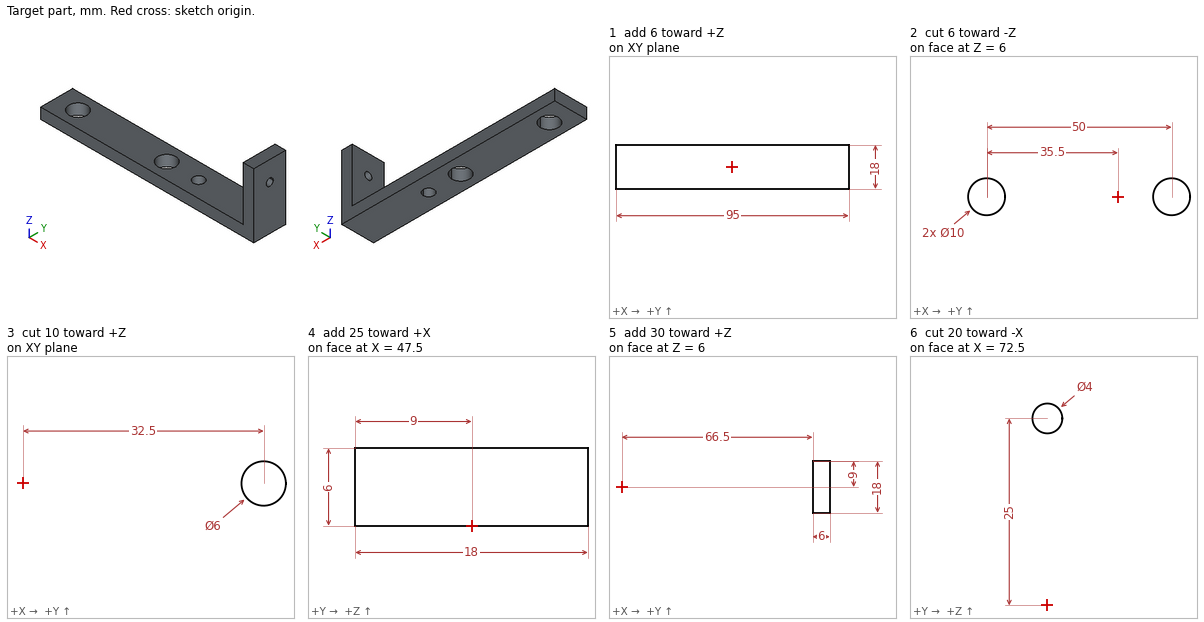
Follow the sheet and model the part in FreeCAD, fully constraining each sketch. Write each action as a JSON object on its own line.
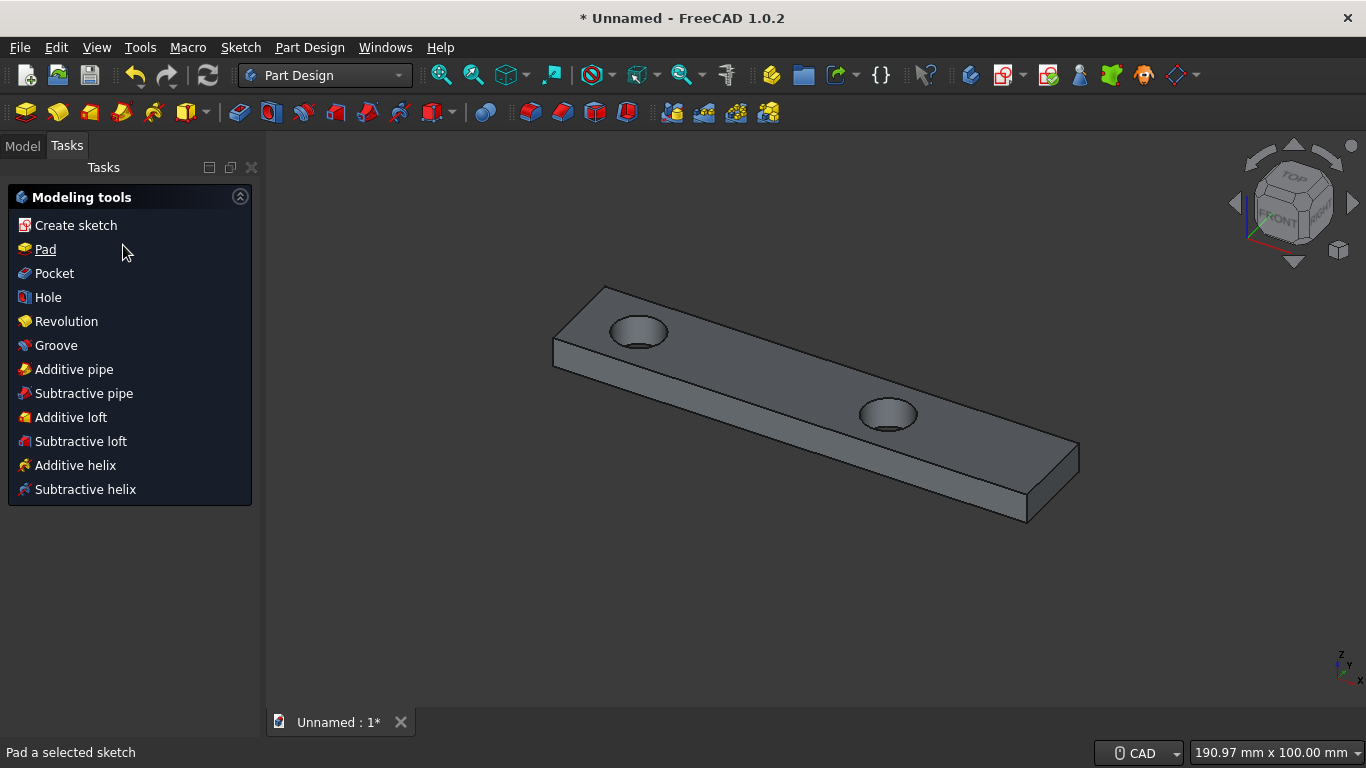
{"action": "left_click", "coordinate": [240, 112]}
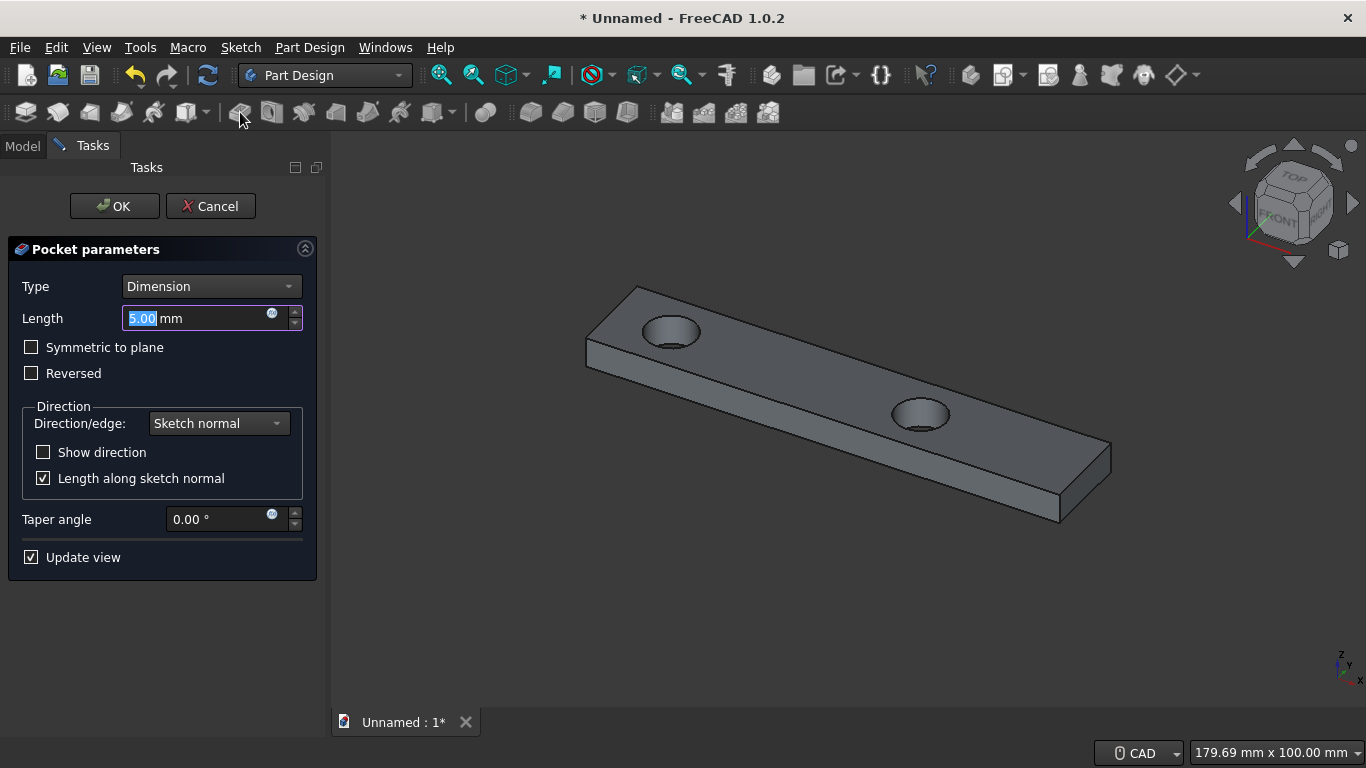
{"action": "type", "text": "10"}
{"action": "key", "text": "Tab"}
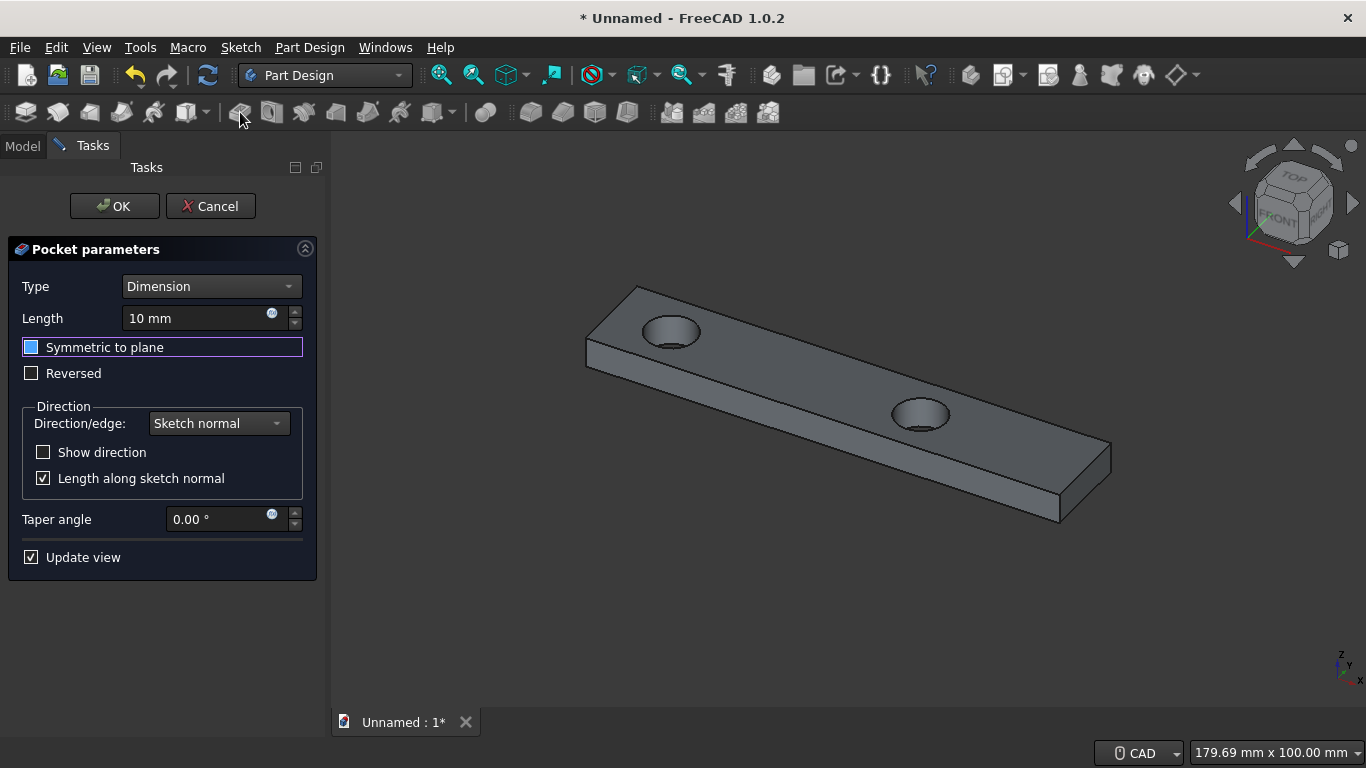
{"action": "left_click", "coordinate": [30, 373]}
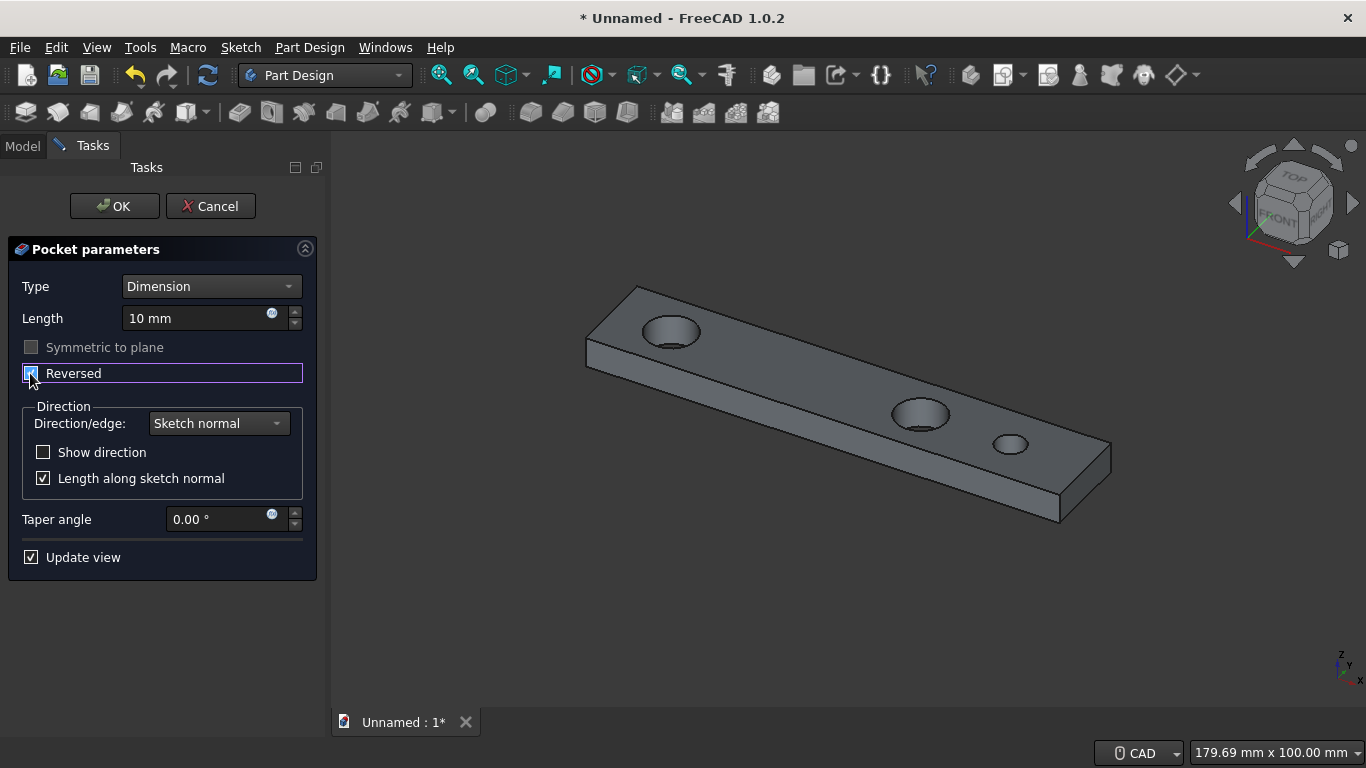
{"action": "left_click", "coordinate": [115, 206]}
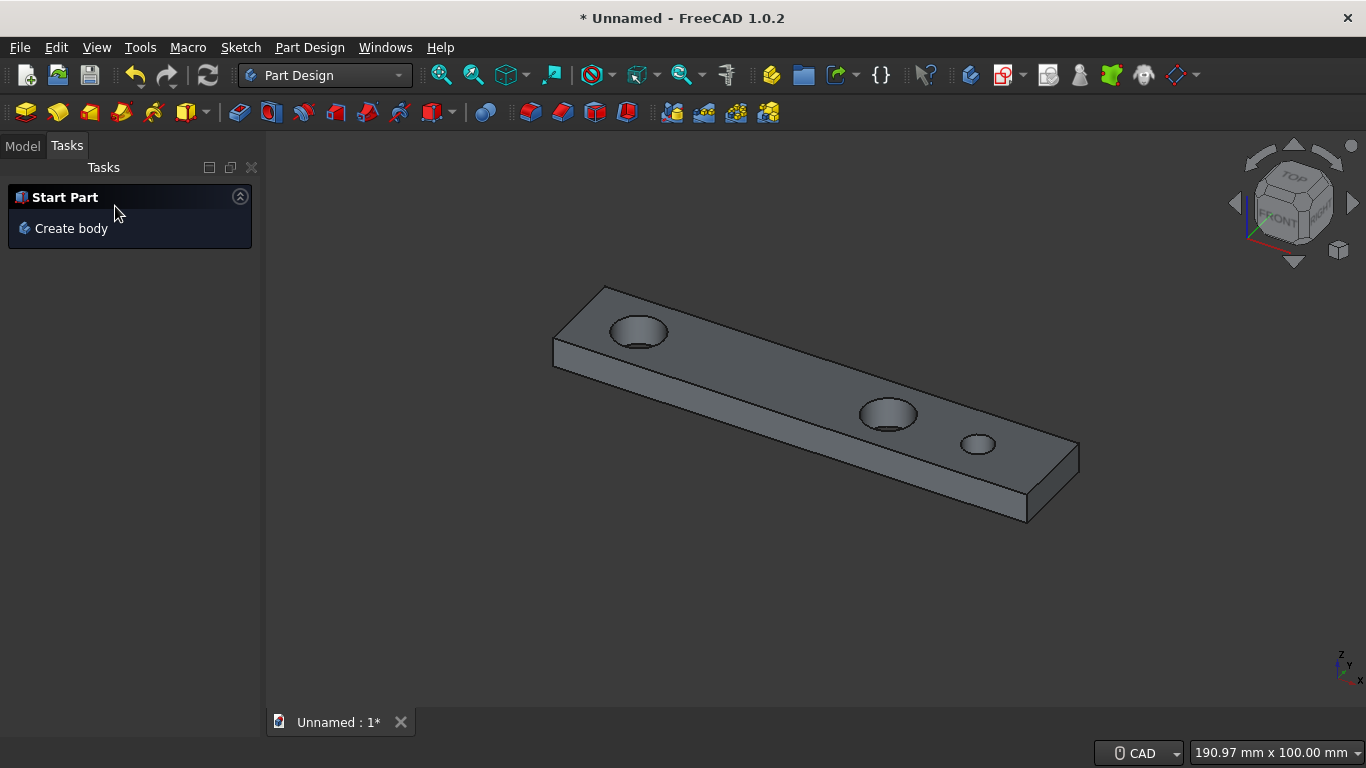
{"action": "left_click", "coordinate": [1068, 468]}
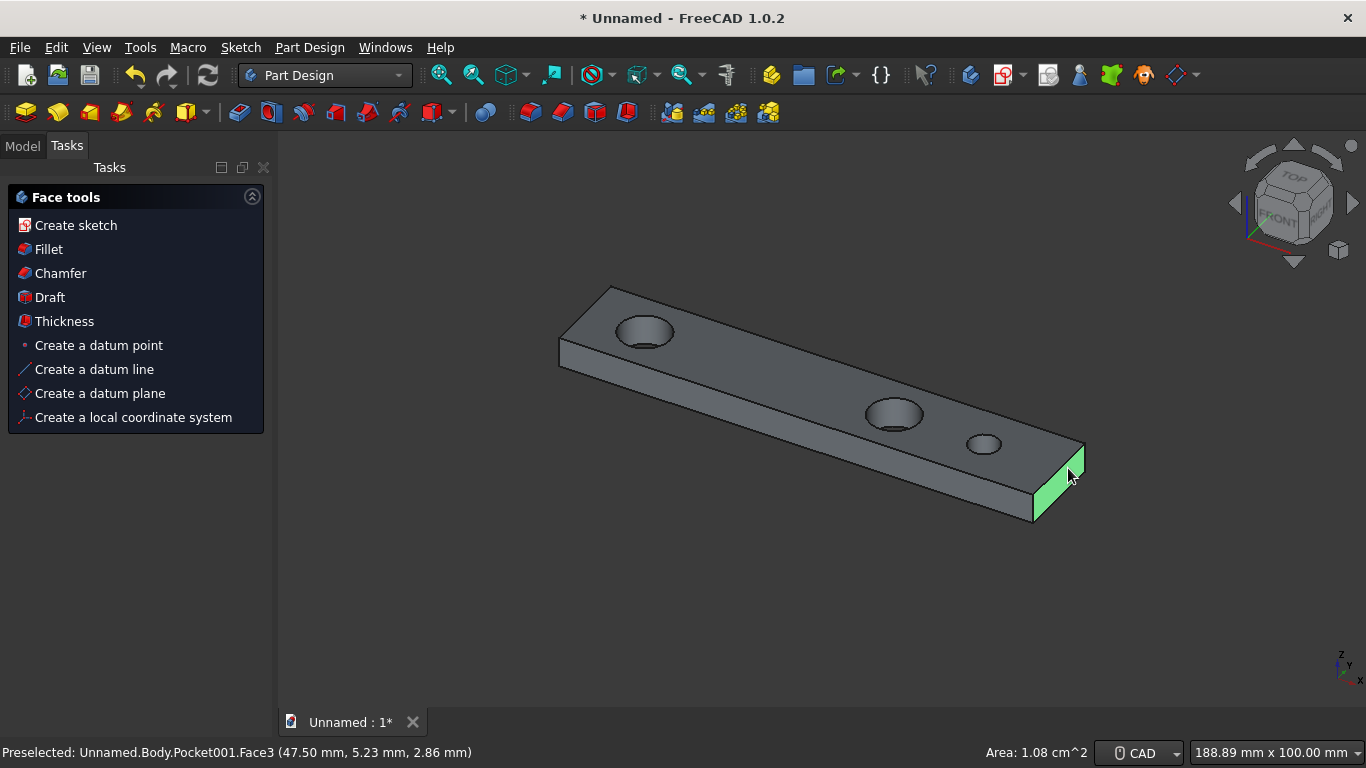
{"action": "left_click", "coordinate": [1004, 76]}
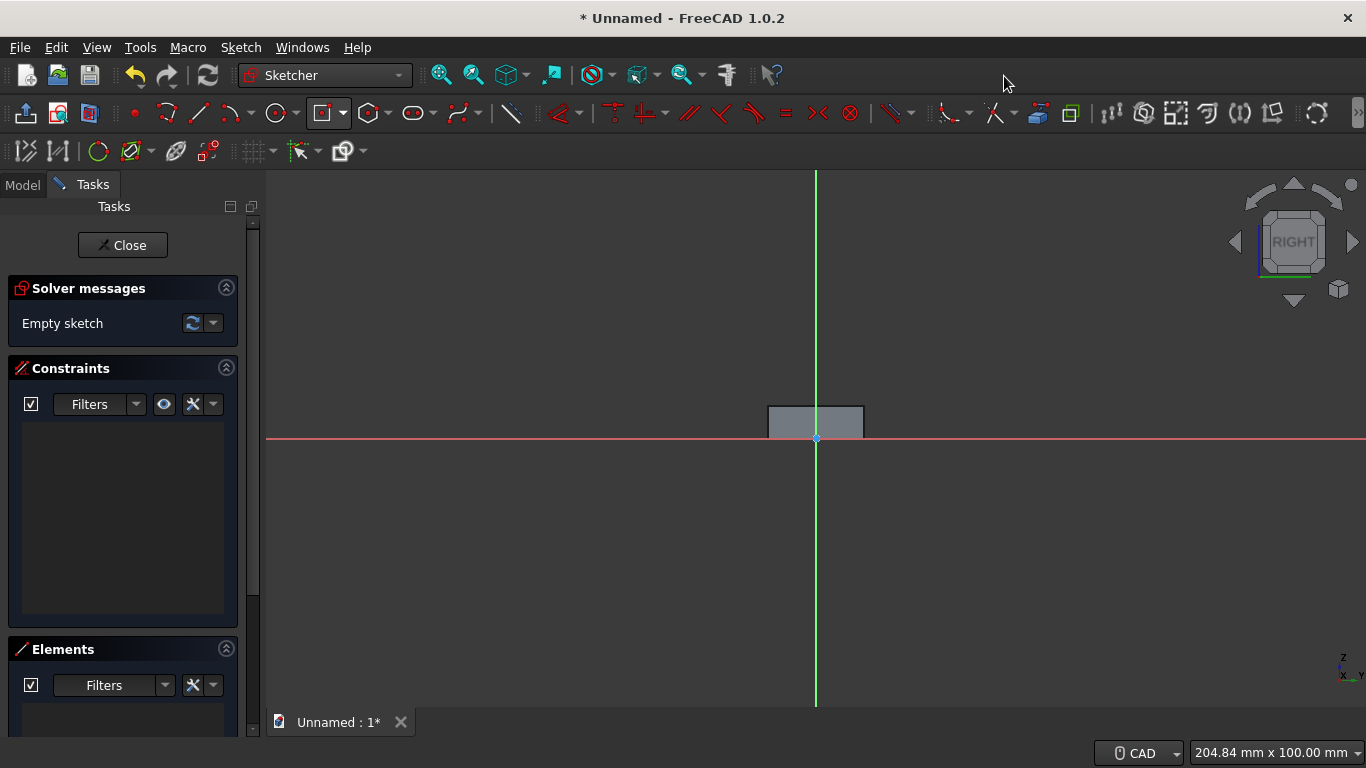
{"action": "scroll", "coordinate": [830, 419], "scroll_direction": "up", "scroll_amount": 9}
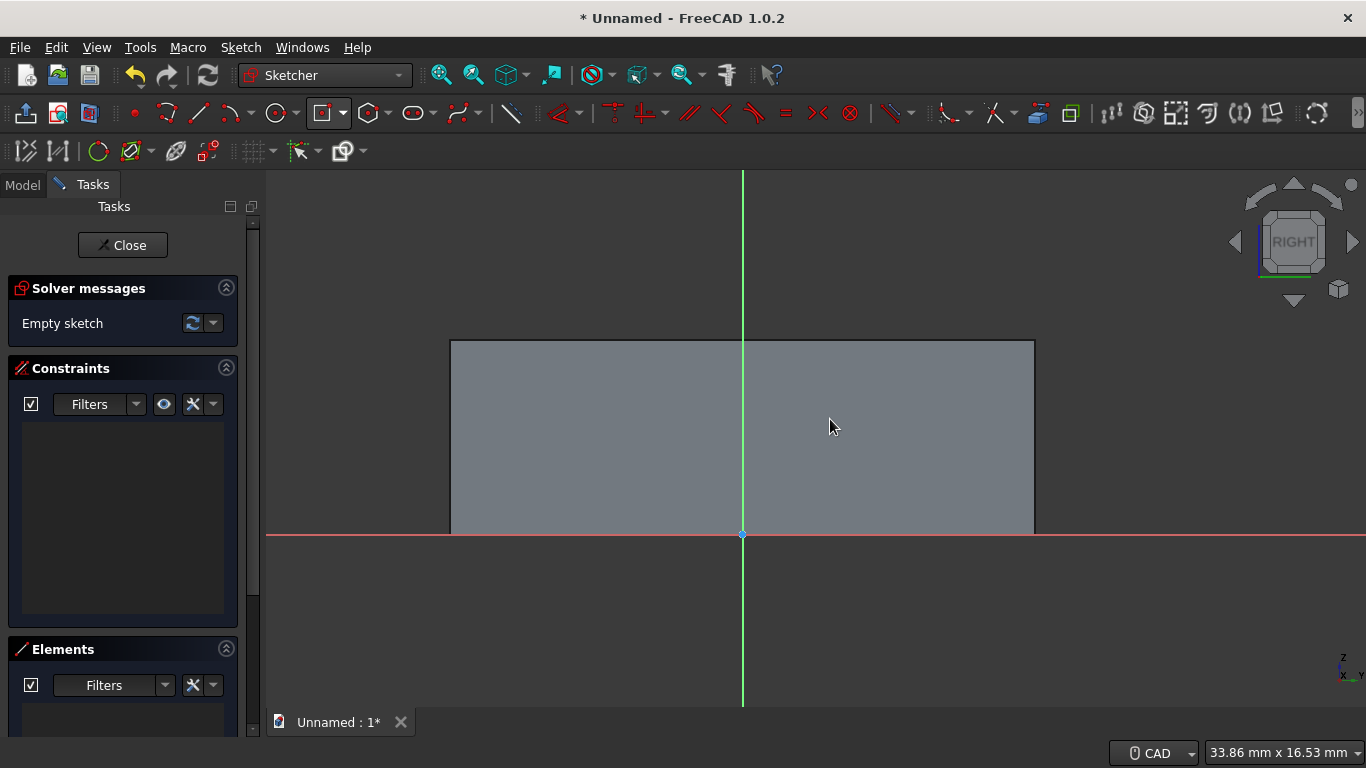
{"action": "left_click", "coordinate": [346, 114]}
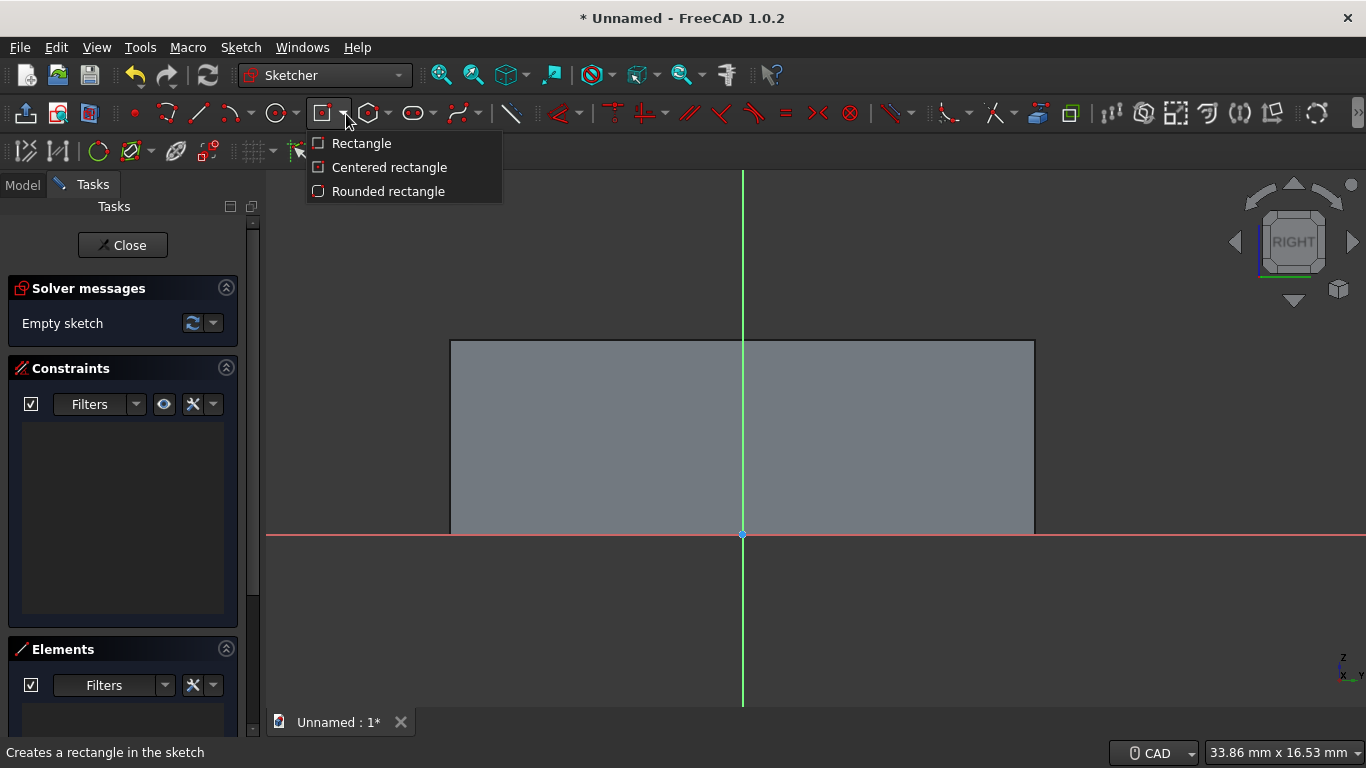
{"action": "left_click", "coordinate": [404, 143]}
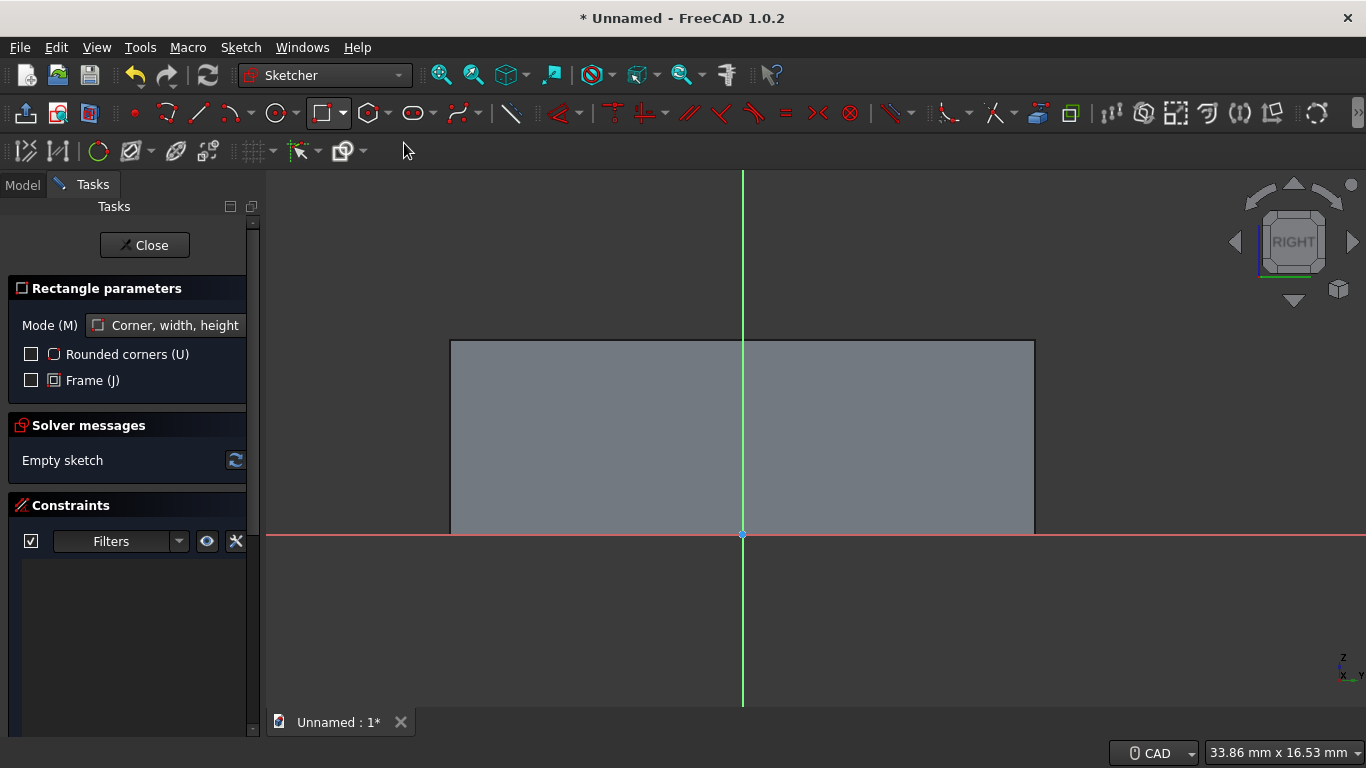
{"action": "left_click", "coordinate": [450, 340]}
{"action": "left_click", "coordinate": [1035, 535]}
{"action": "key", "text": "Escape"}